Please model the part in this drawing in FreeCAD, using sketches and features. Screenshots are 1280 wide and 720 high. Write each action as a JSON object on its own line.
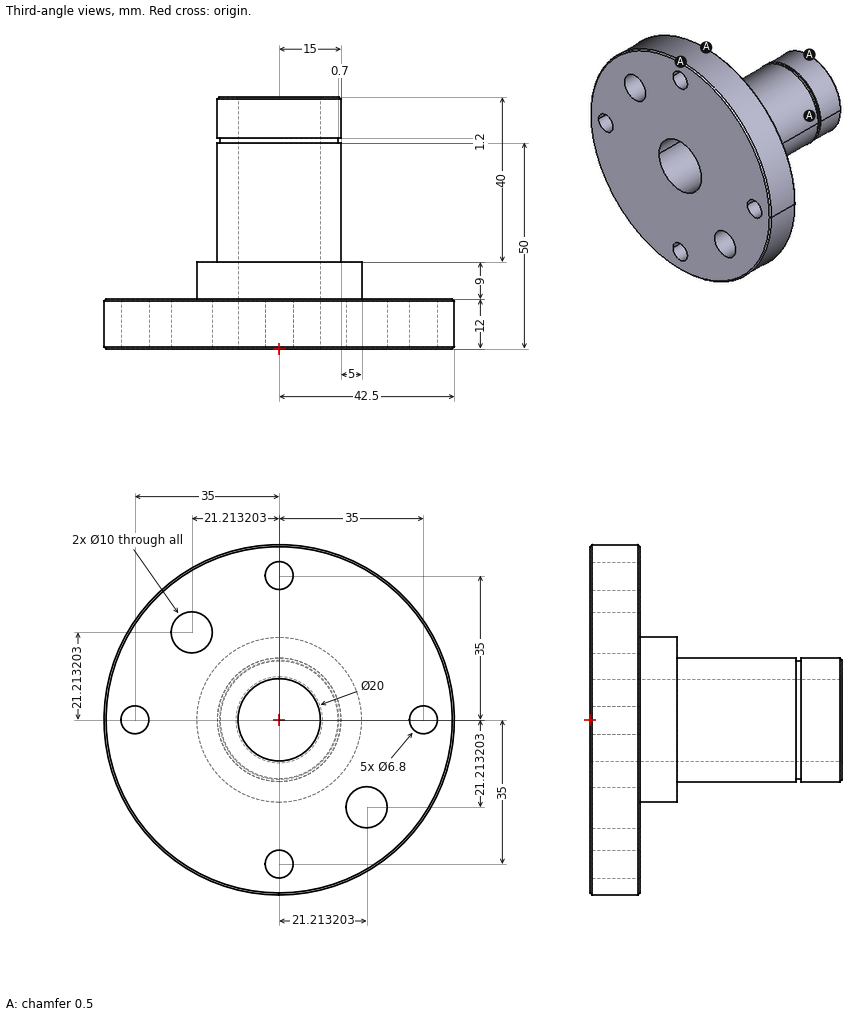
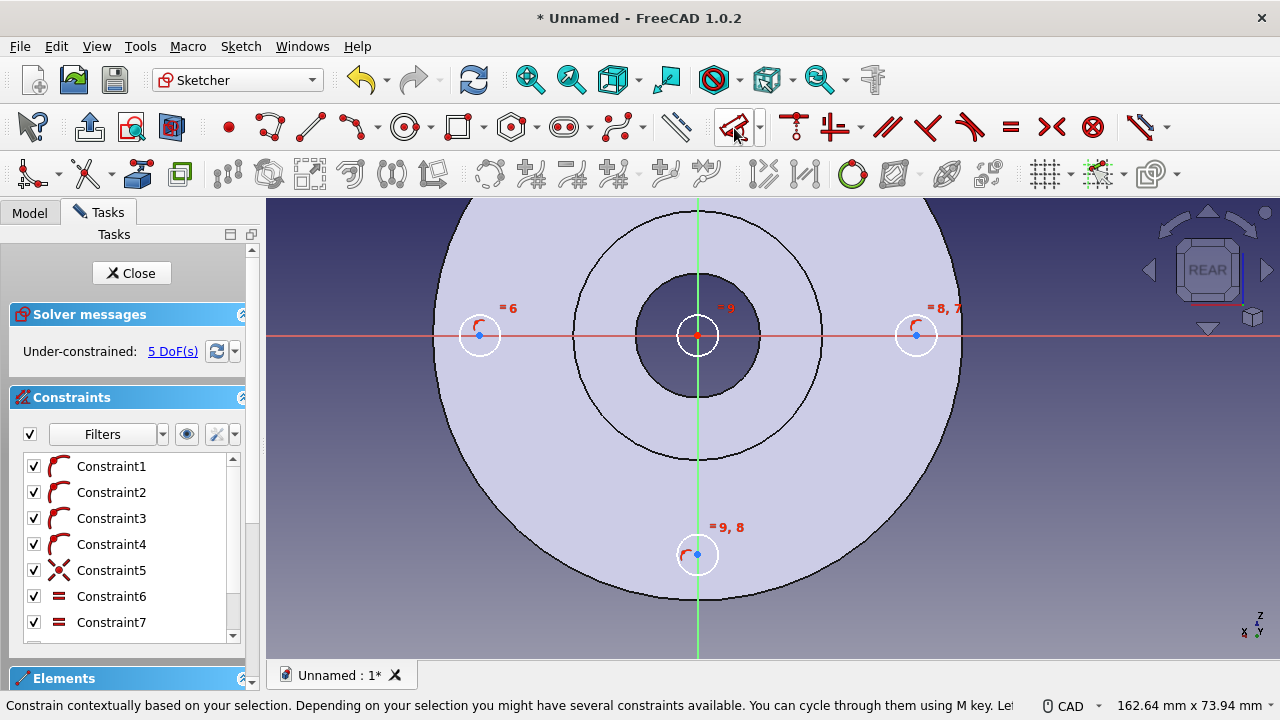
{"action": "left_click", "coordinate": [494, 321]}
{"action": "left_click", "coordinate": [516, 298]}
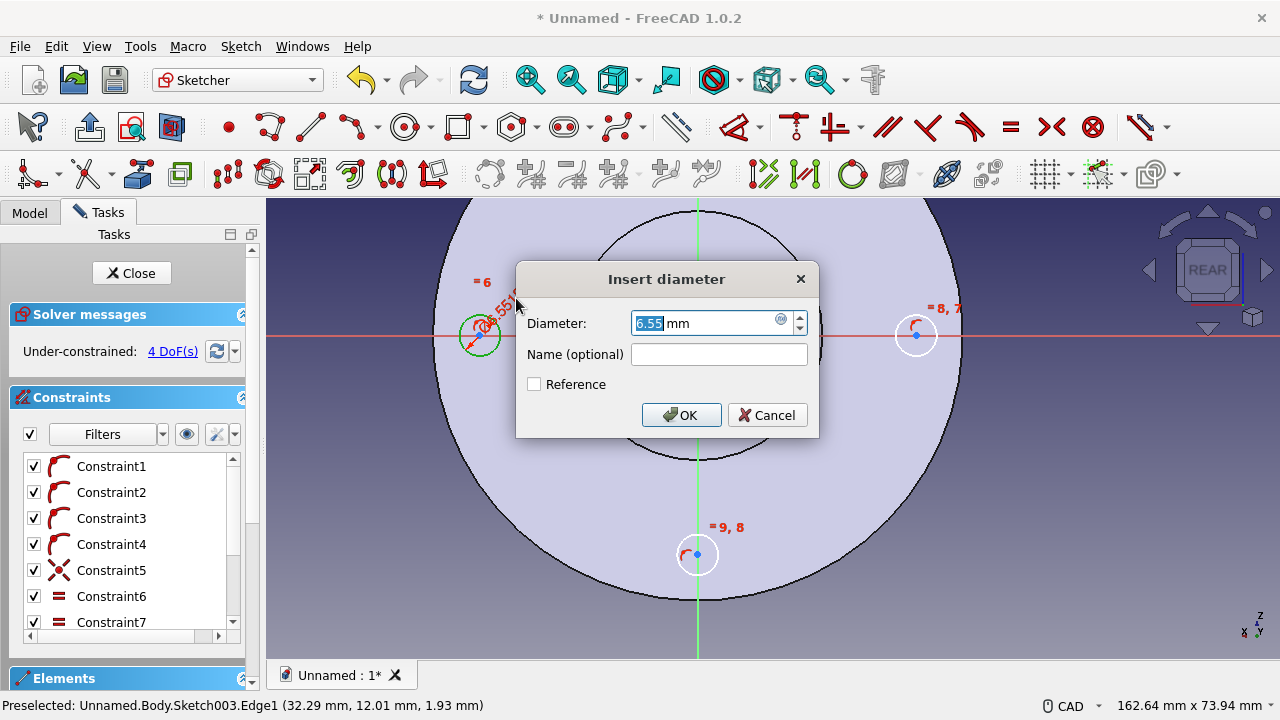
{"action": "type", "text": "6.8"}
{"action": "key", "text": "Return"}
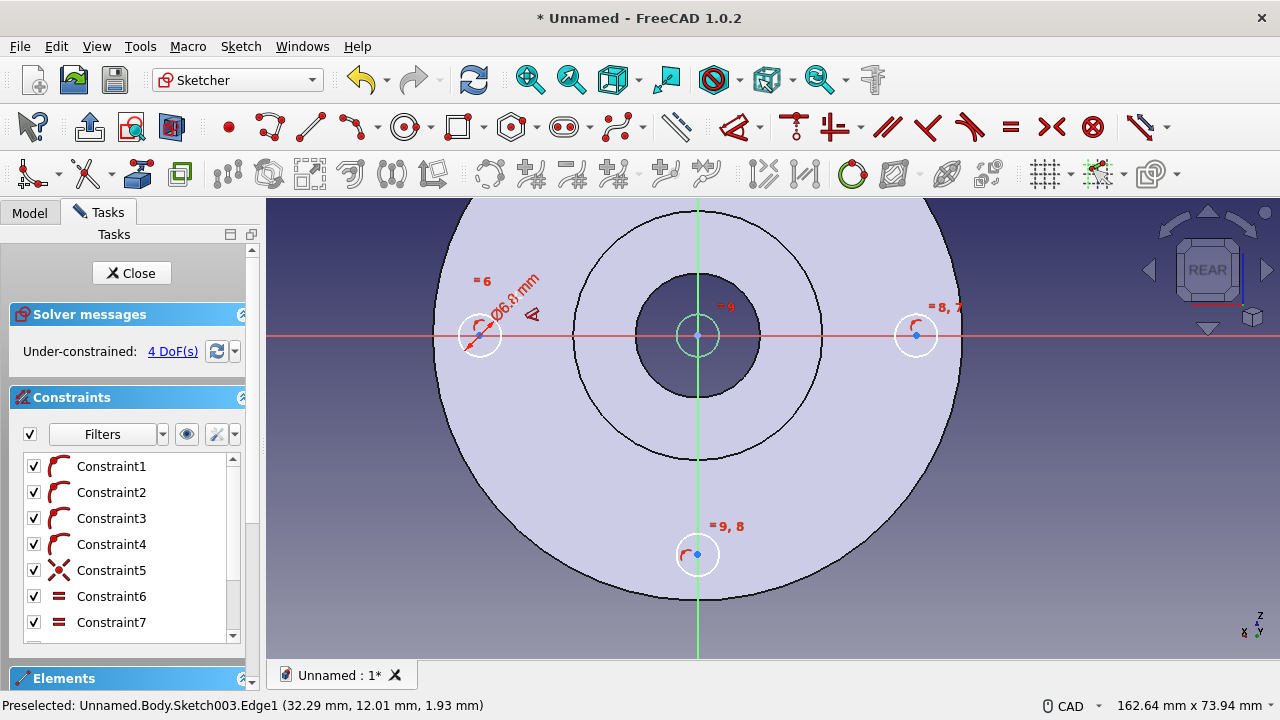
{"action": "left_click", "coordinate": [480, 336]}
{"action": "left_click", "coordinate": [589, 370]}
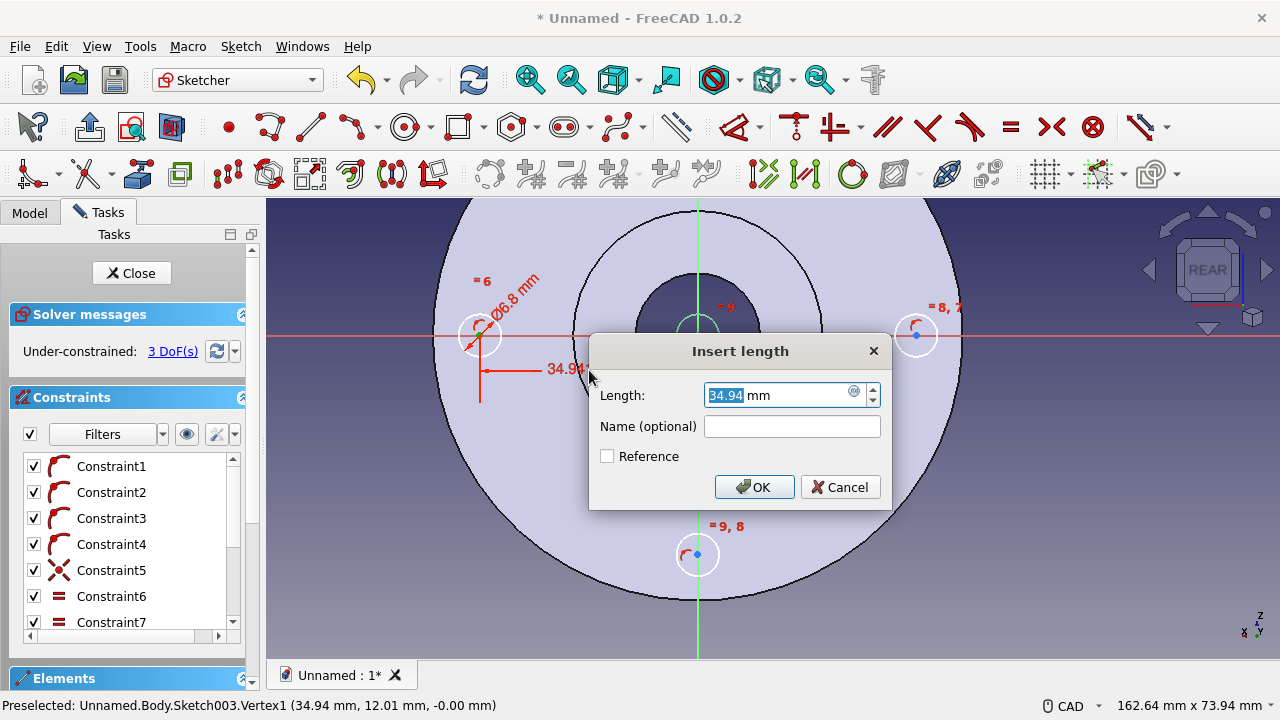
{"action": "type", "text": "35"}
{"action": "key", "text": "Return"}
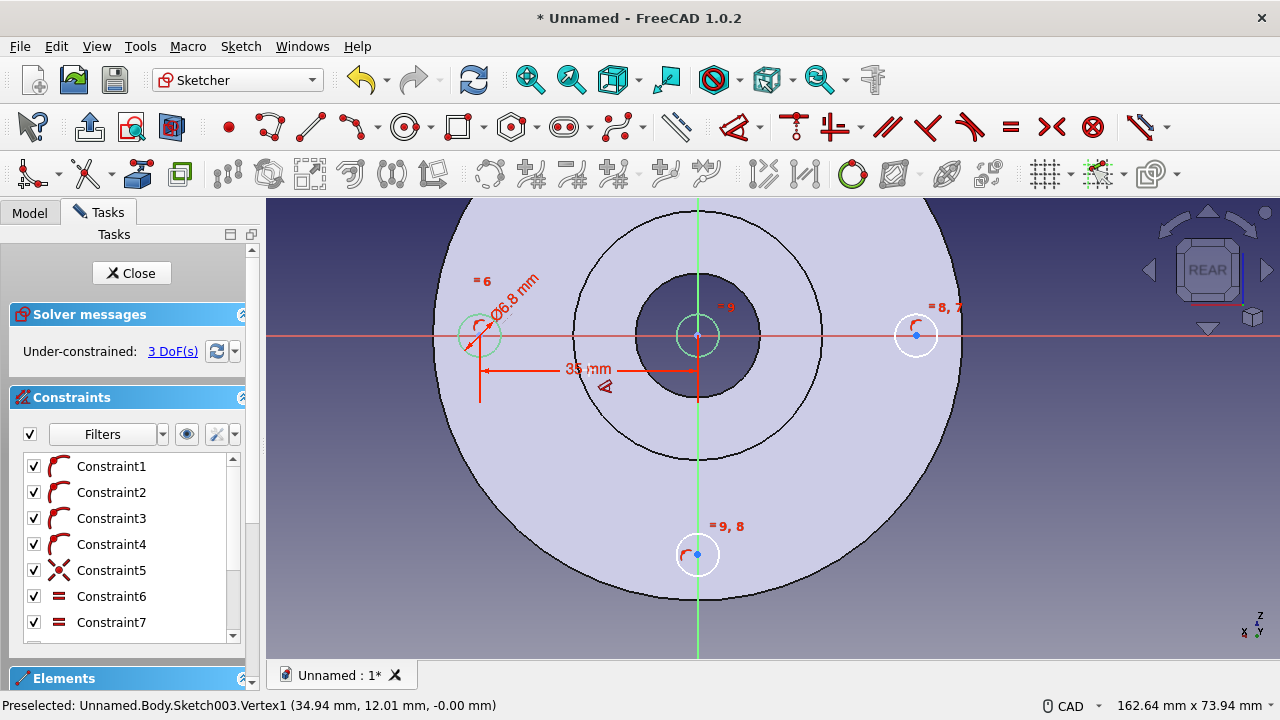
{"action": "scroll", "coordinate": [713, 542], "scroll_direction": "down", "scroll_amount": 3}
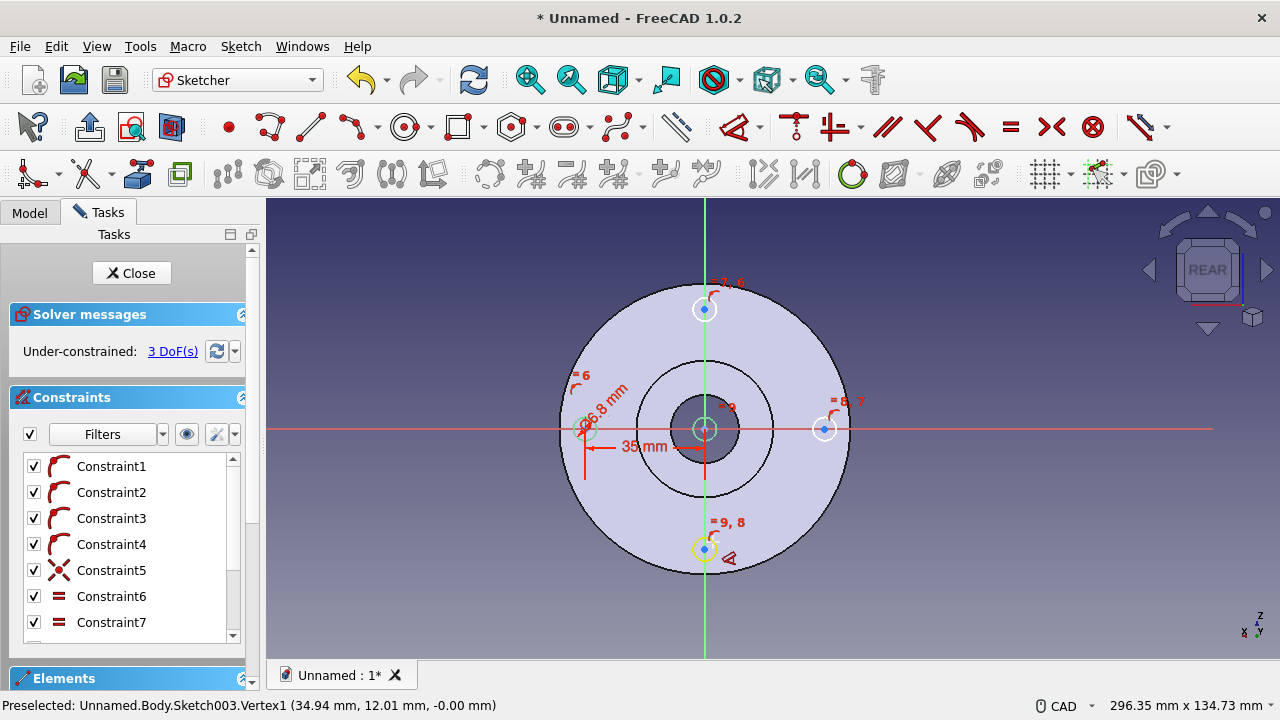
{"action": "left_click", "coordinate": [705, 310]}
{"action": "left_click", "coordinate": [739, 369]}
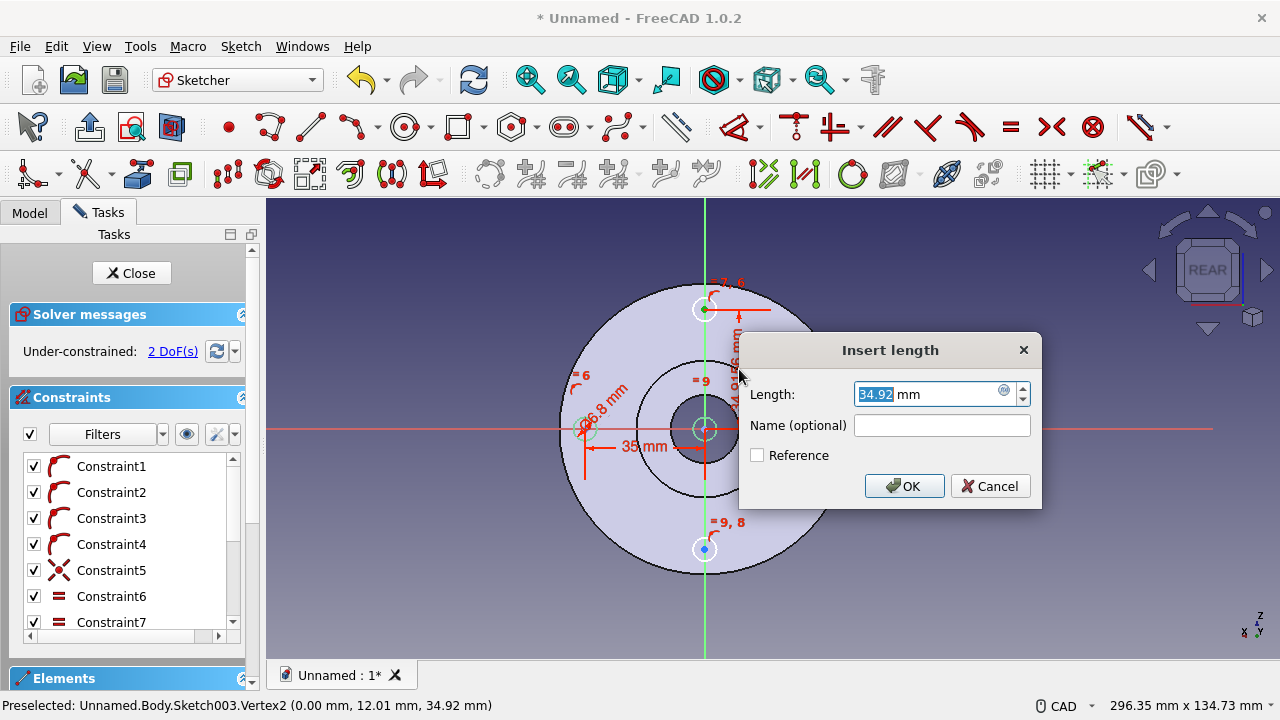
{"action": "type", "text": "35"}
{"action": "key", "text": "Return"}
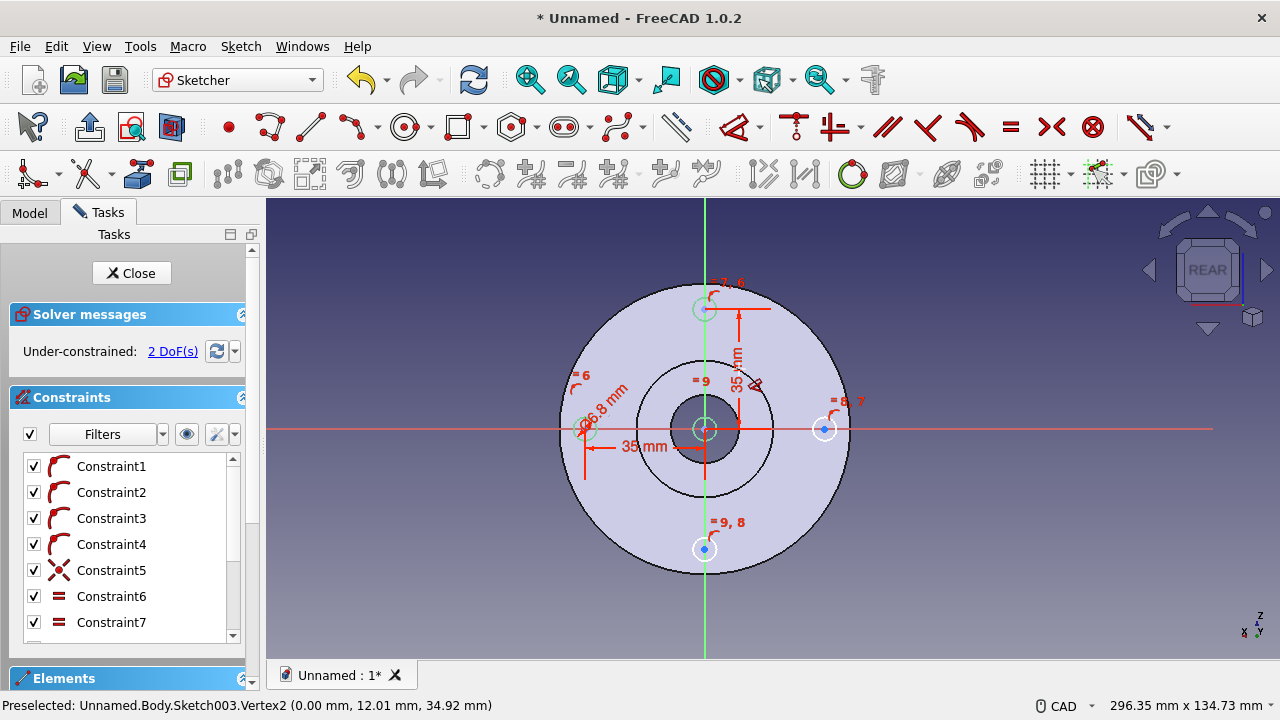
{"action": "left_click", "coordinate": [825, 429]}
{"action": "left_click", "coordinate": [765, 463]}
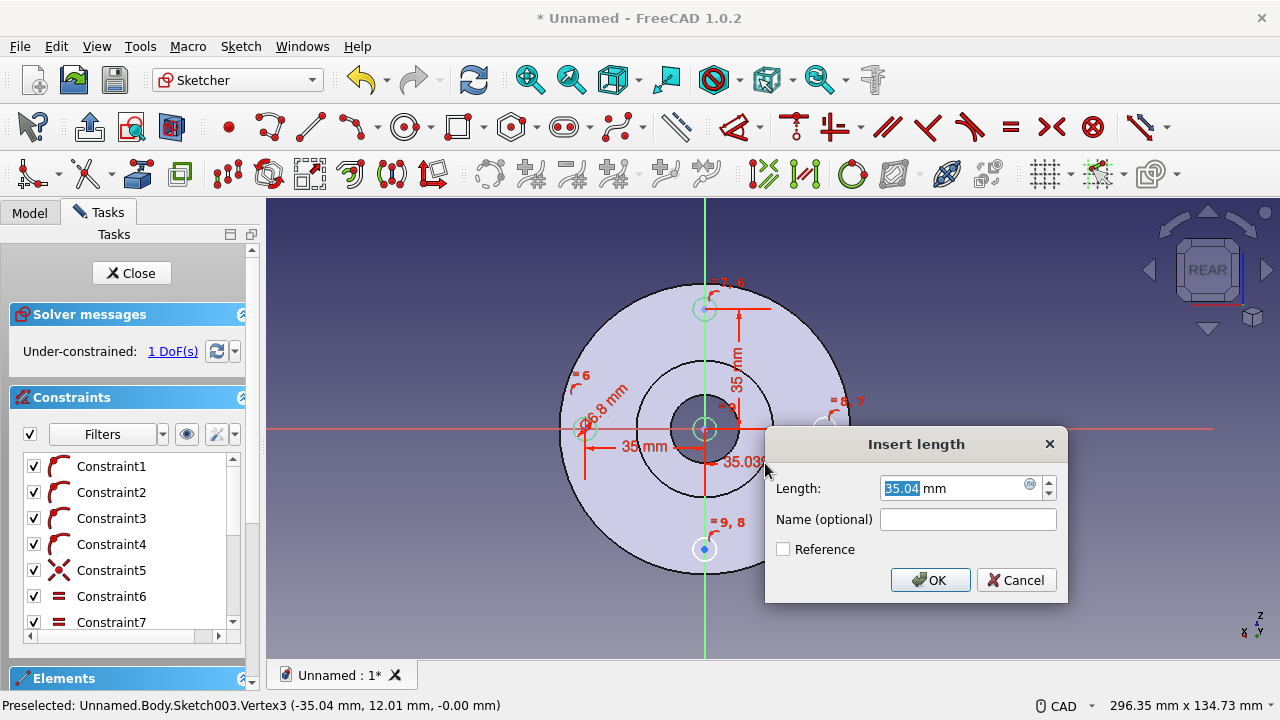
{"action": "type", "text": "35"}
{"action": "key", "text": "Return"}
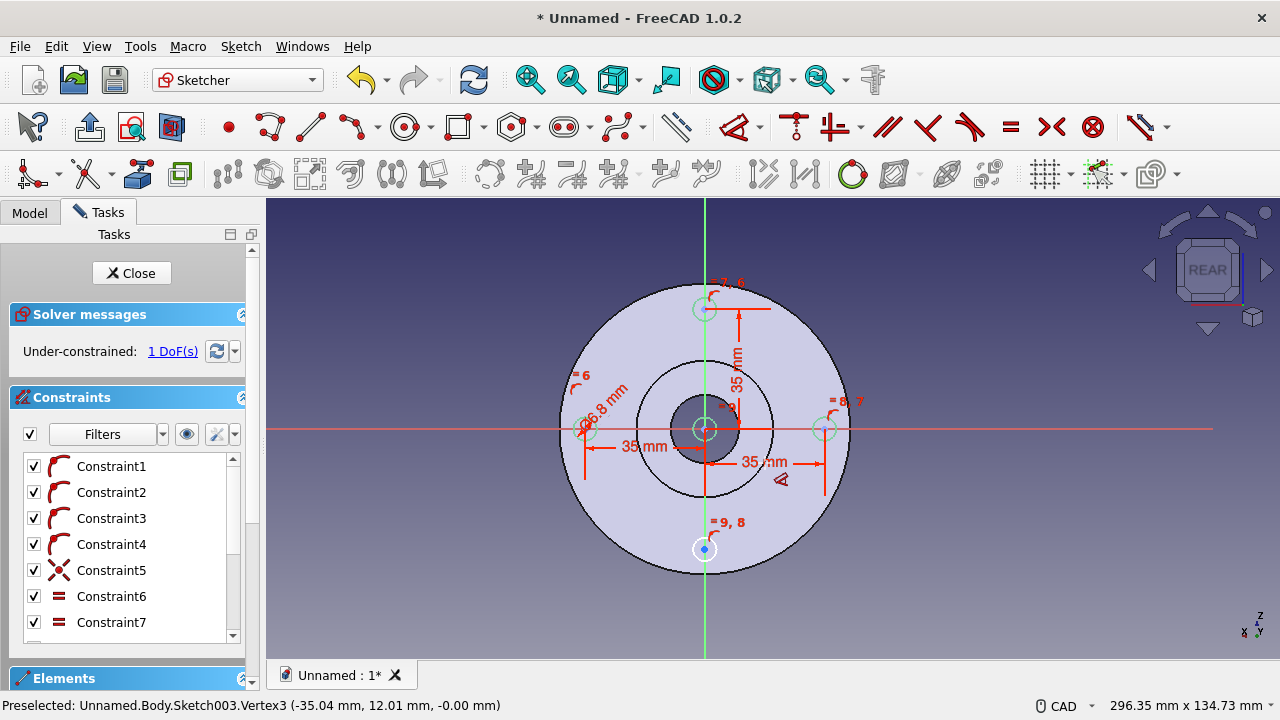
{"action": "left_click", "coordinate": [705, 549]}
{"action": "left_click", "coordinate": [739, 489]}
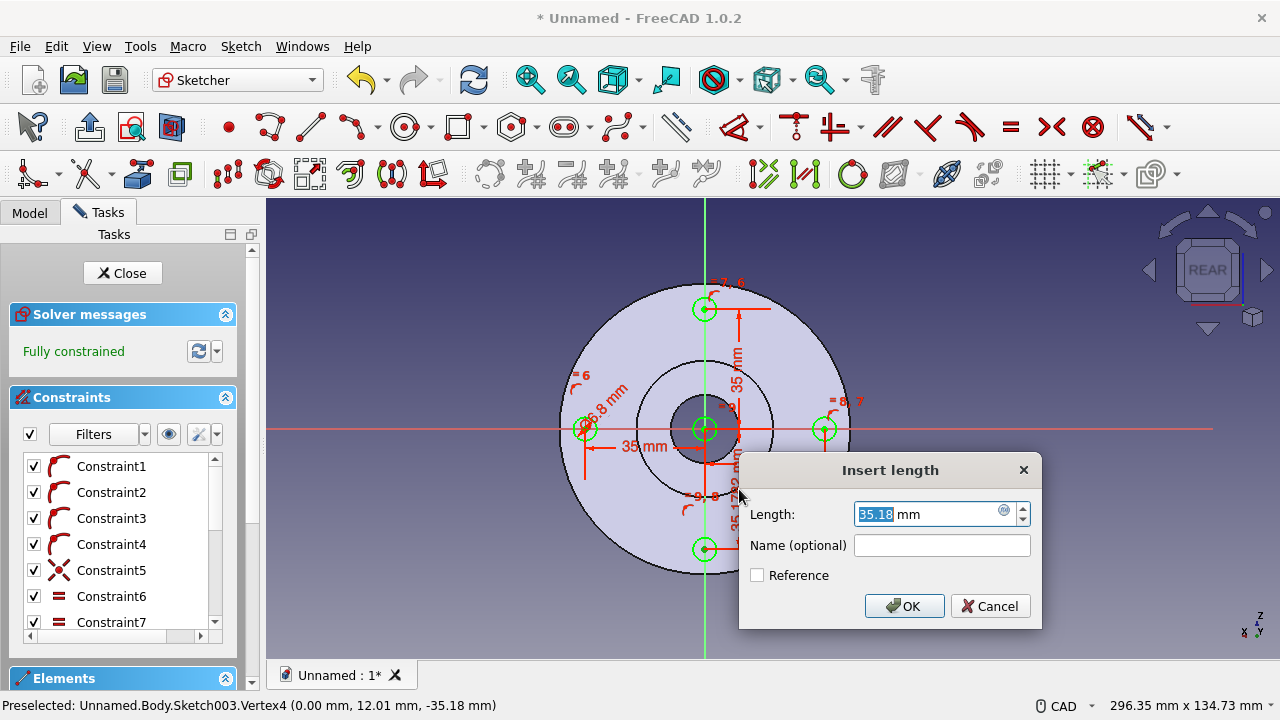
{"action": "type", "text": "35"}
{"action": "key", "text": "Return"}
{"action": "key", "text": "Escape"}